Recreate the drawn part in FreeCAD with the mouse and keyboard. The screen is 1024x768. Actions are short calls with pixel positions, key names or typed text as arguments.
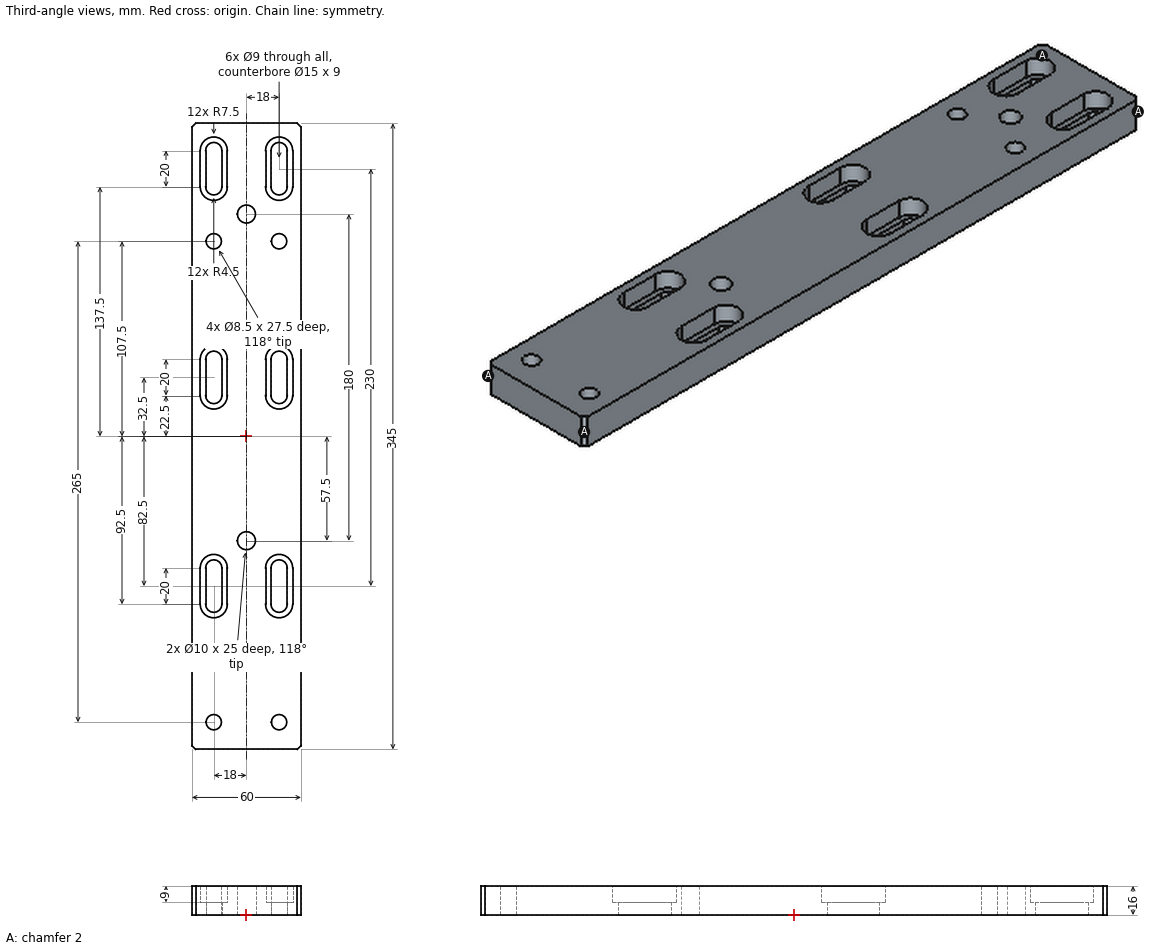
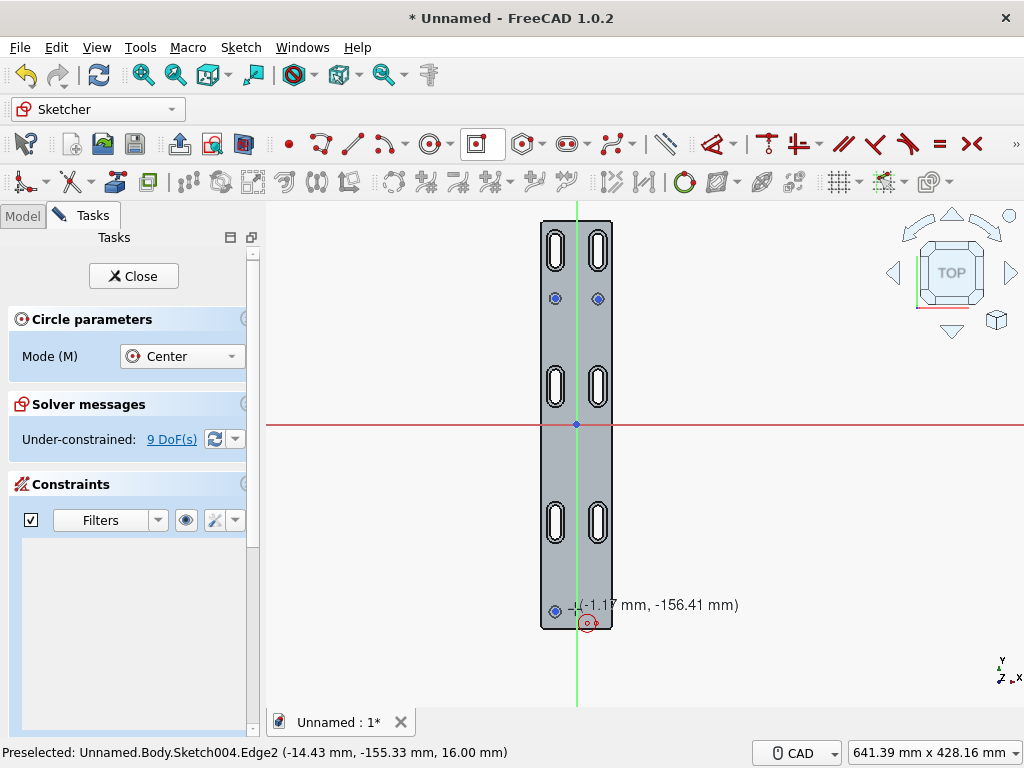
click(598, 611)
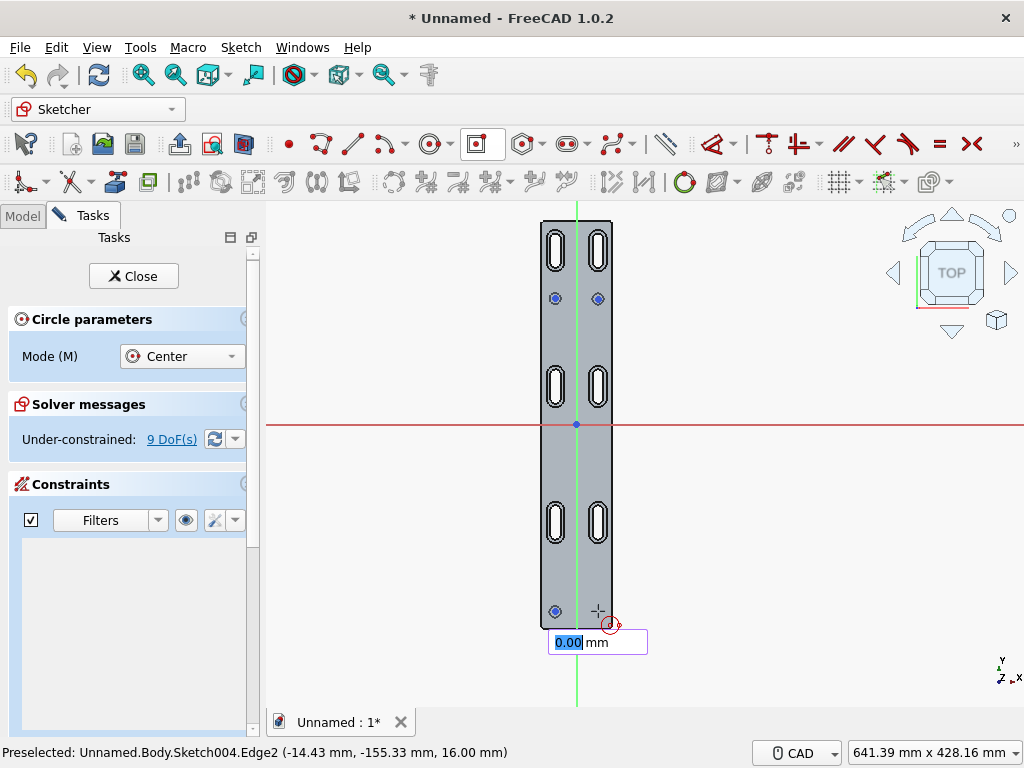
scroll(602, 608, up, 6)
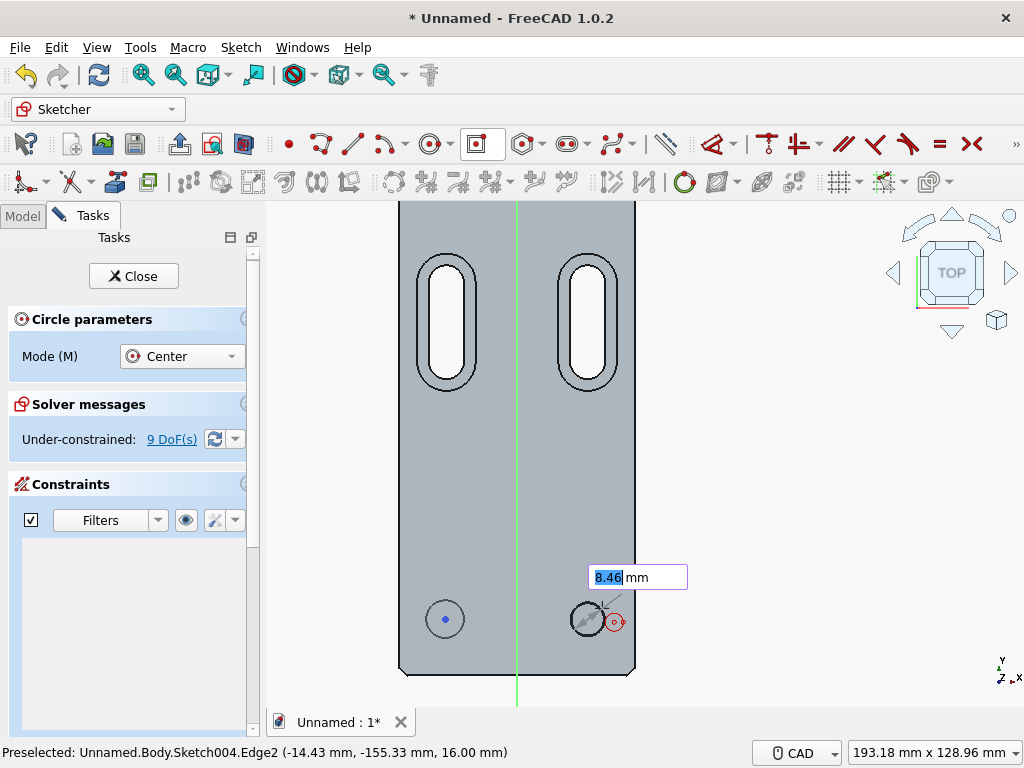
click(599, 605)
key(Escape)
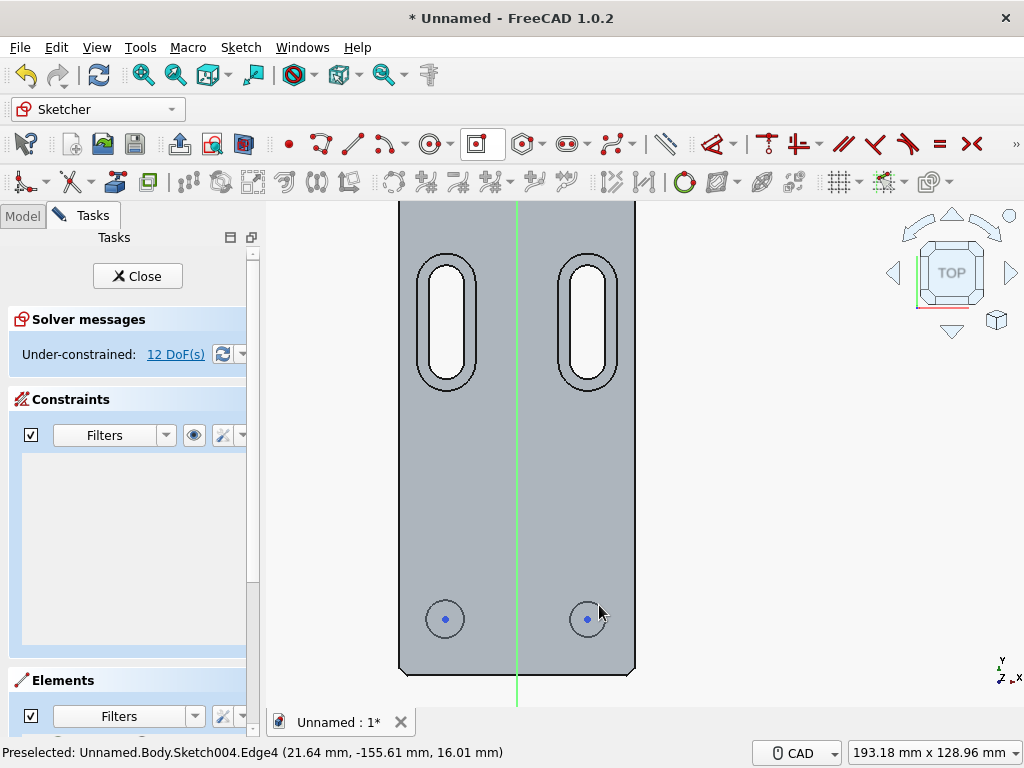
scroll(602, 608, down, 6)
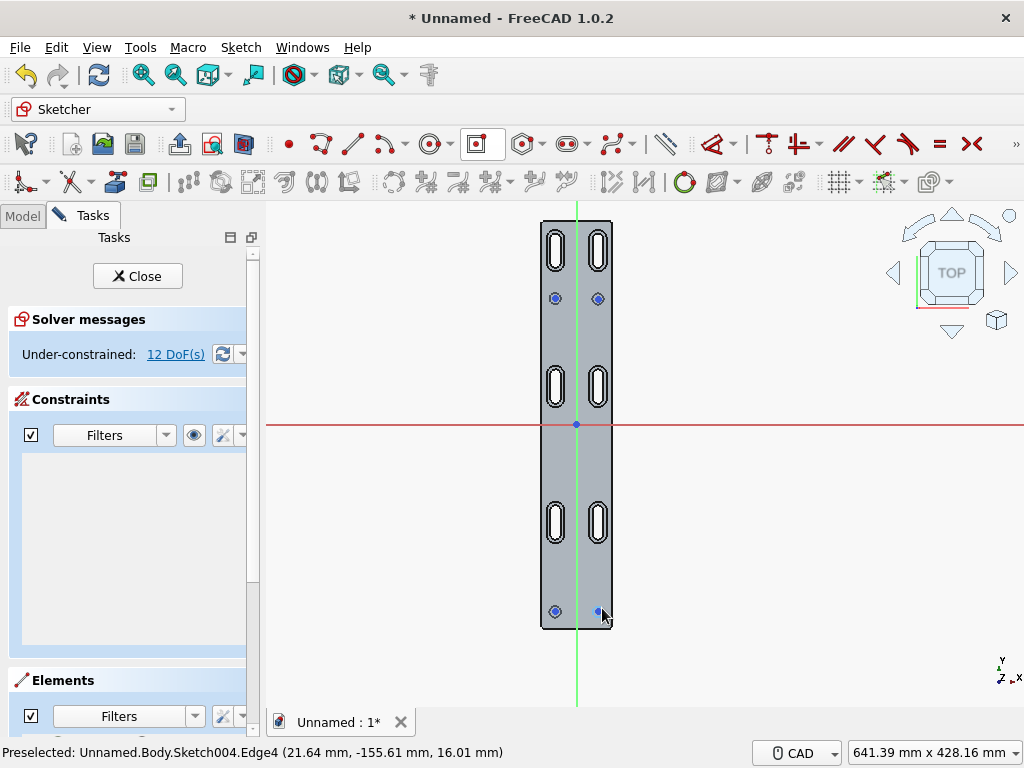
scroll(559, 295, up, 5)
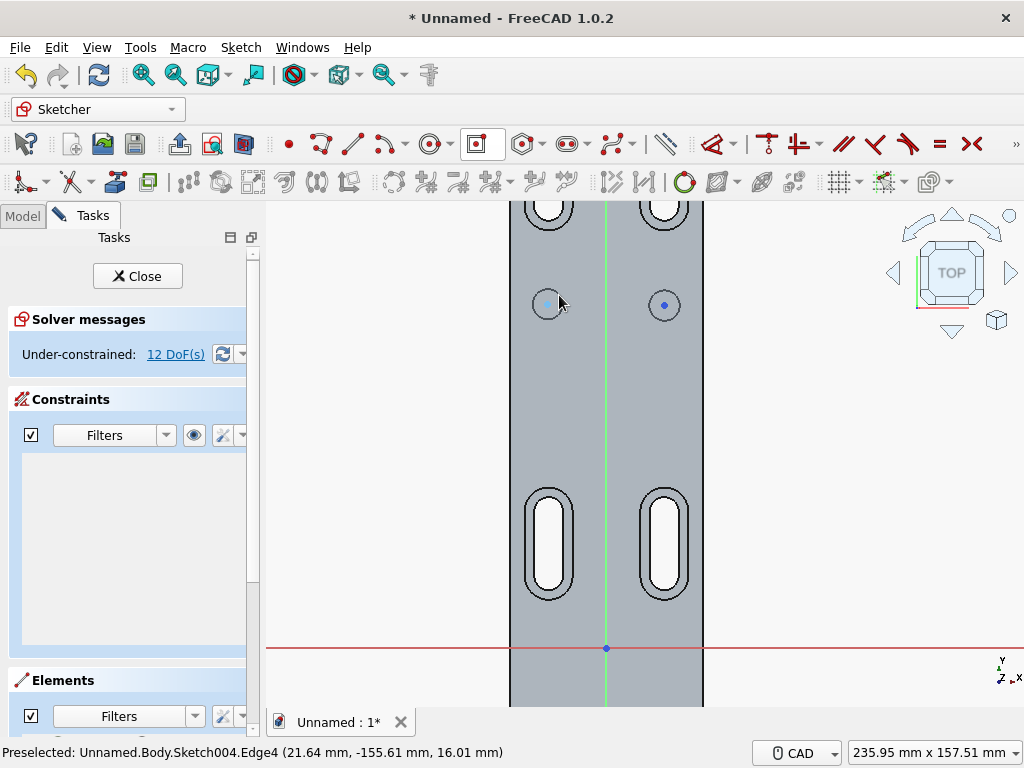
click(558, 294)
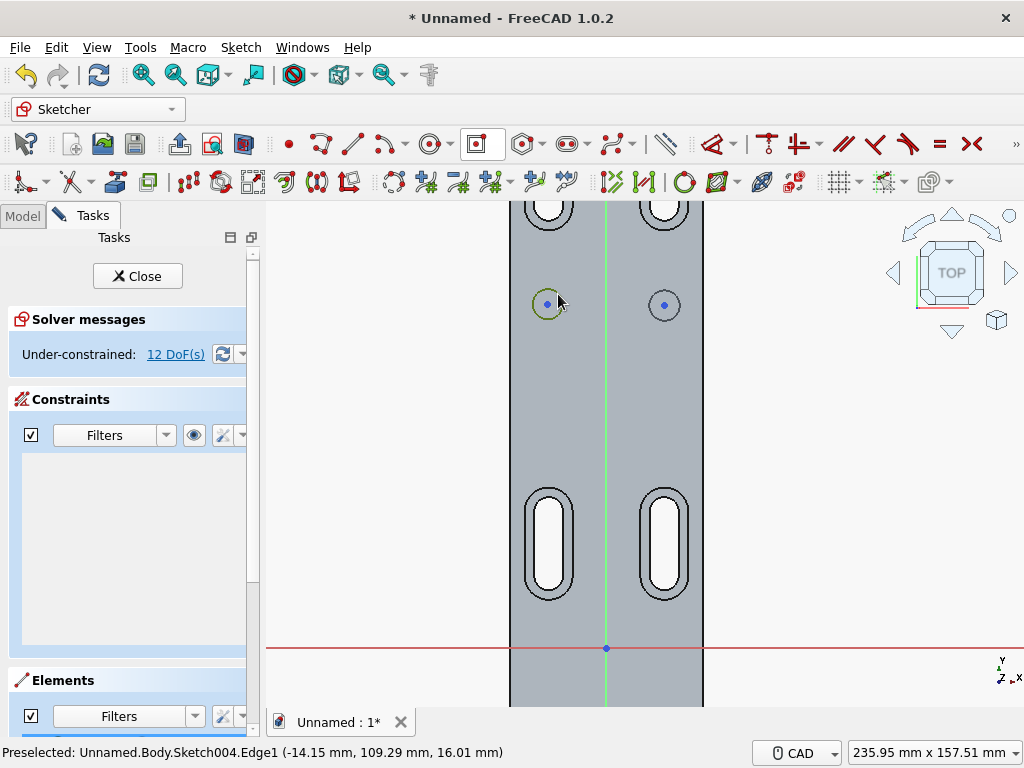
click(675, 295)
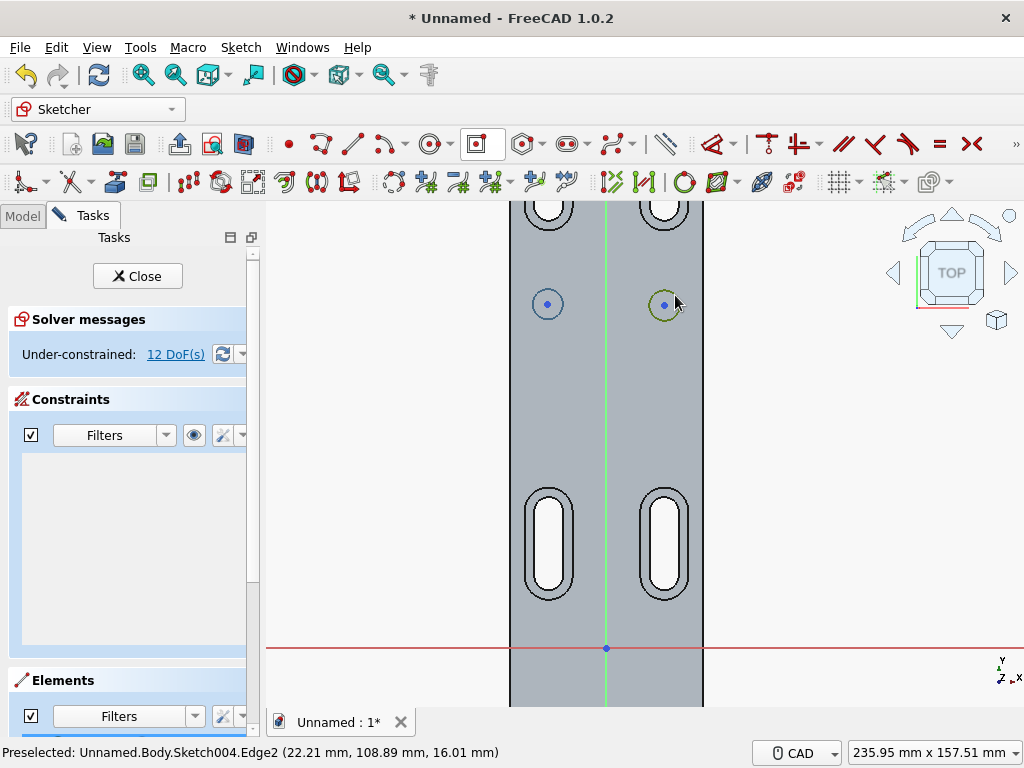
scroll(559, 294, down, 5)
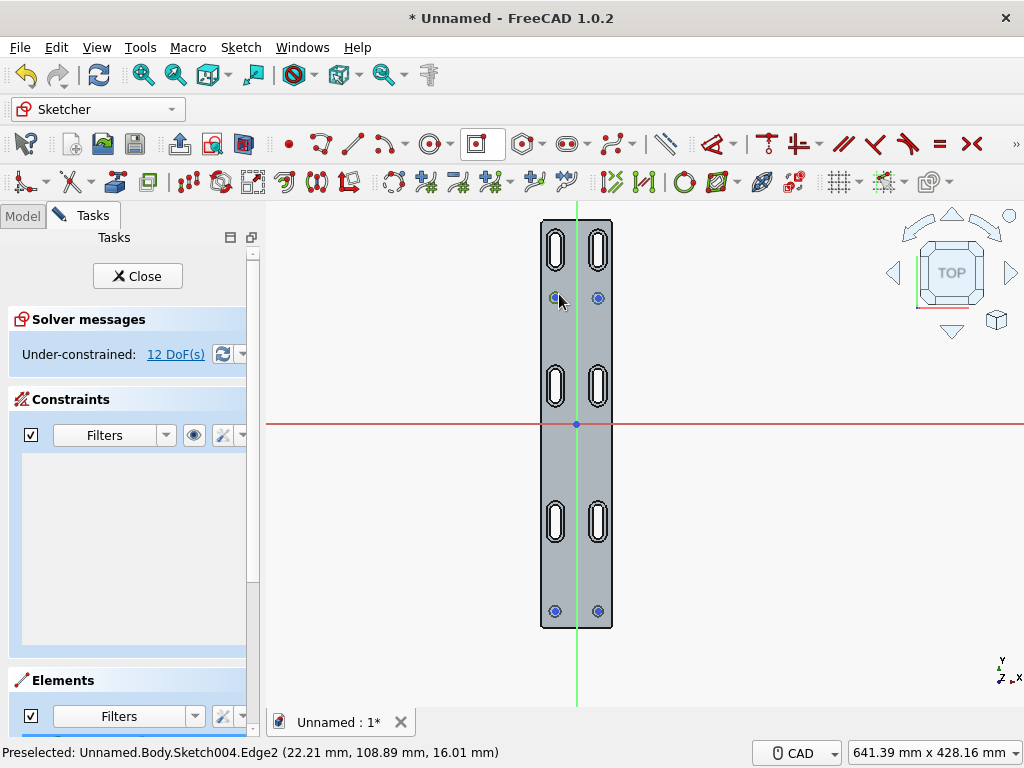
scroll(559, 607, up, 5)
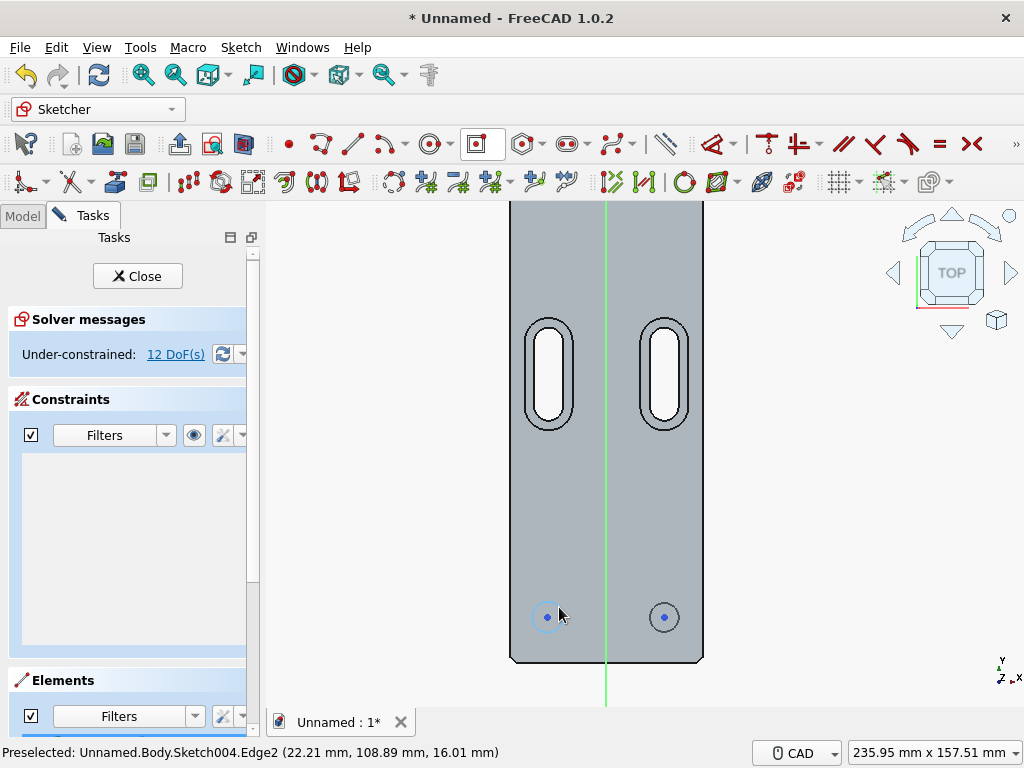
click(558, 606)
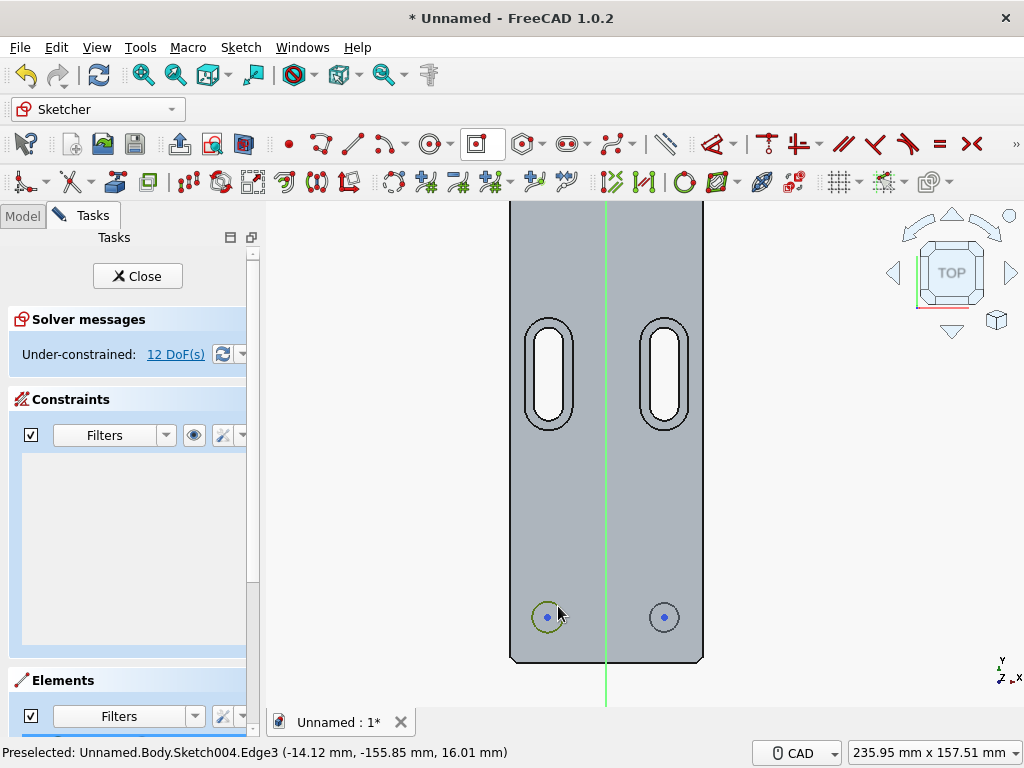
click(674, 607)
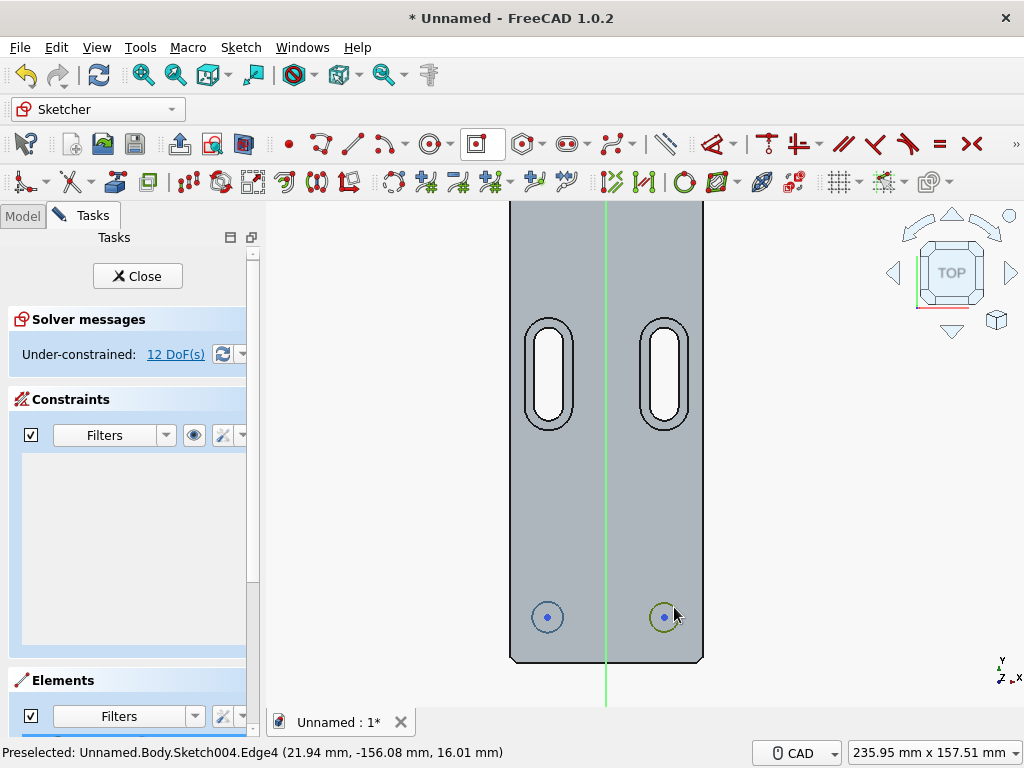
key(e)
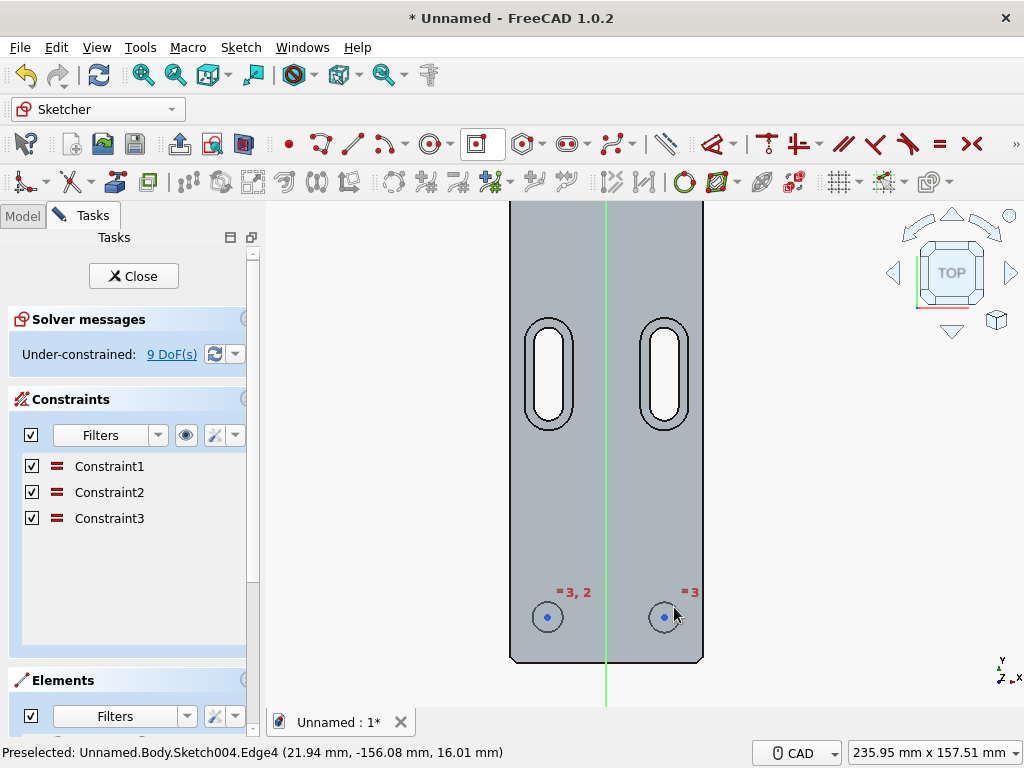
scroll(559, 608, down, 5)